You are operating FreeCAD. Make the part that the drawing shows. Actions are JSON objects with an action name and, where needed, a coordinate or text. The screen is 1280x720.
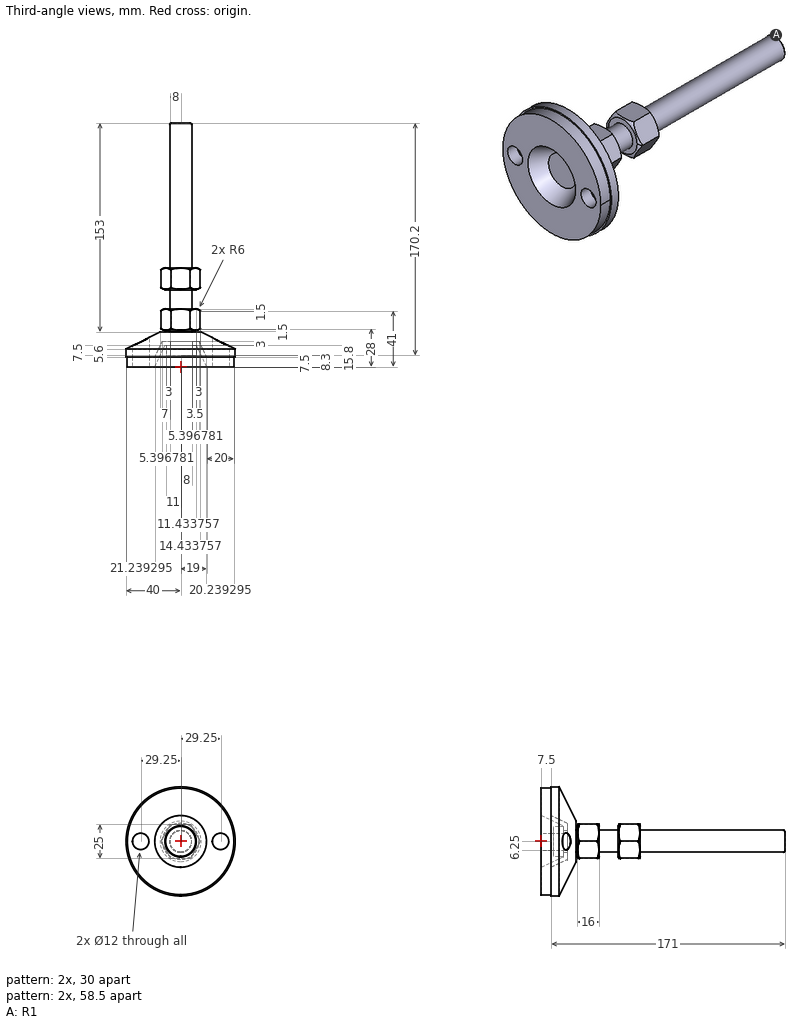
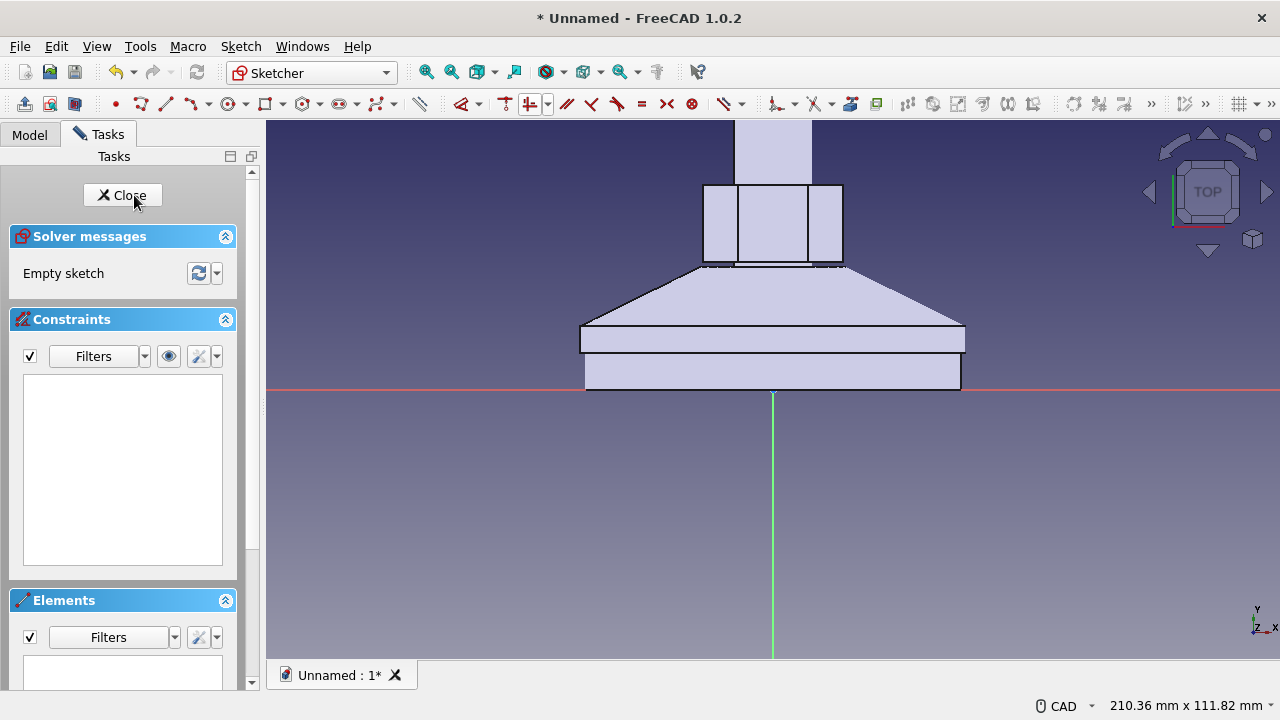
{"action": "left_click", "coordinate": [75, 104]}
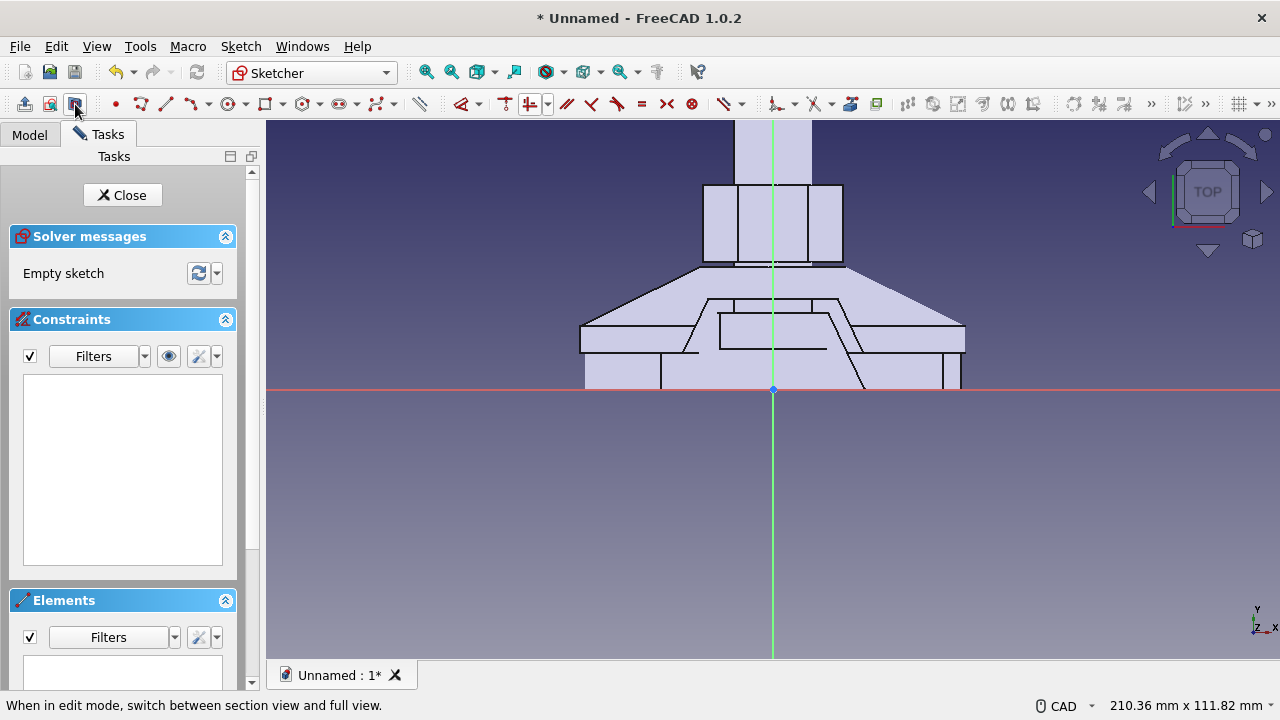
{"action": "scroll", "coordinate": [878, 169], "scroll_direction": "up", "scroll_amount": 7}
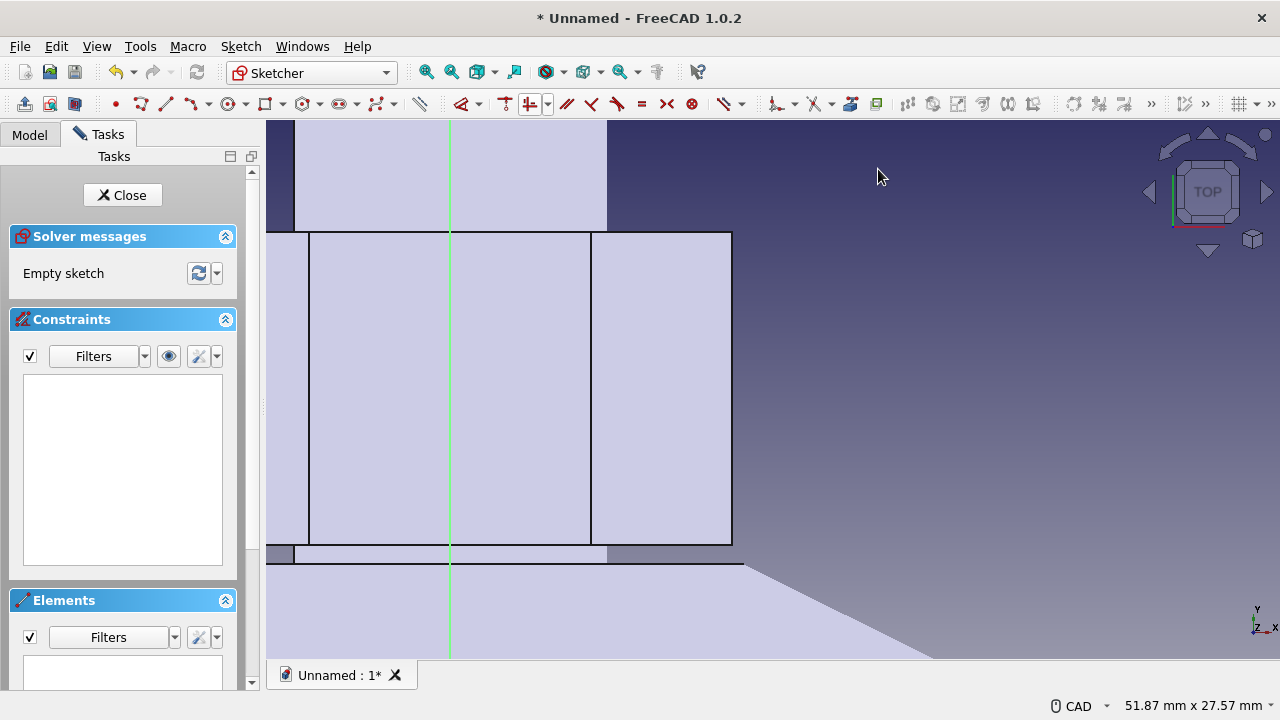
{"action": "left_click", "coordinate": [141, 104]}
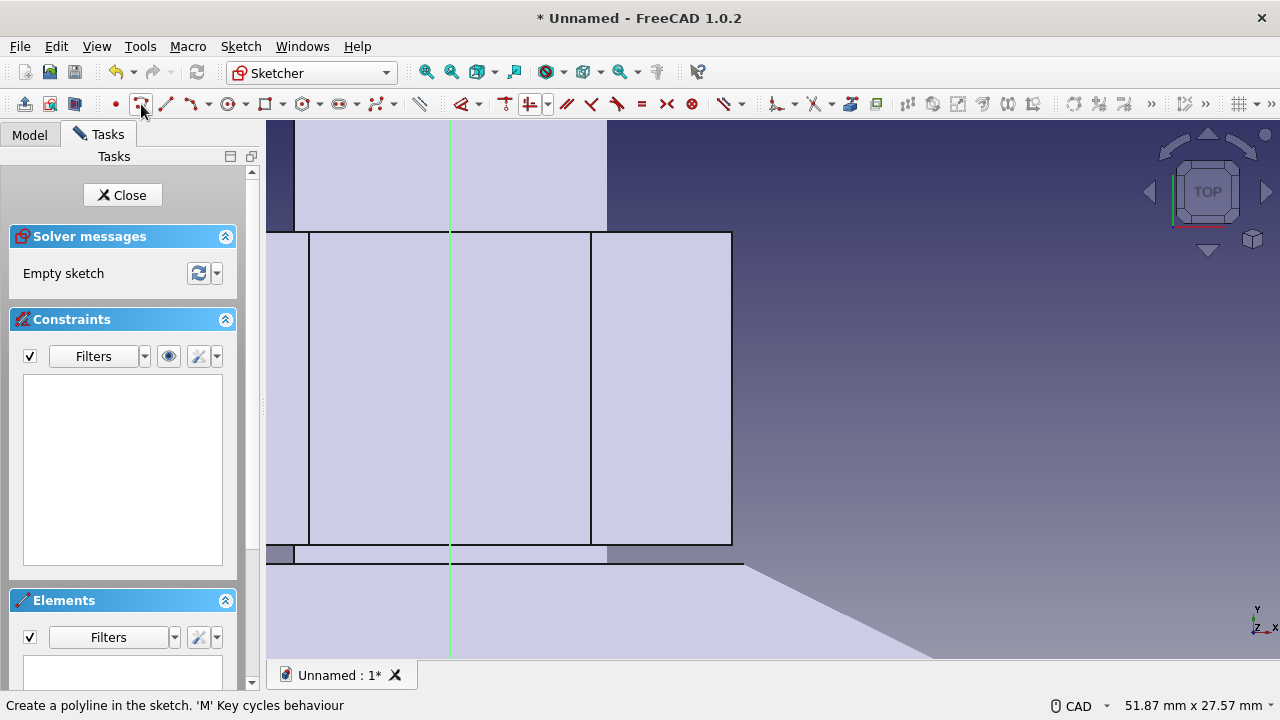
{"action": "left_click", "coordinate": [732, 261]}
{"action": "left_click", "coordinate": [732, 232]}
{"action": "left_click", "coordinate": [674, 232]}
{"action": "right_click", "coordinate": [674, 232]}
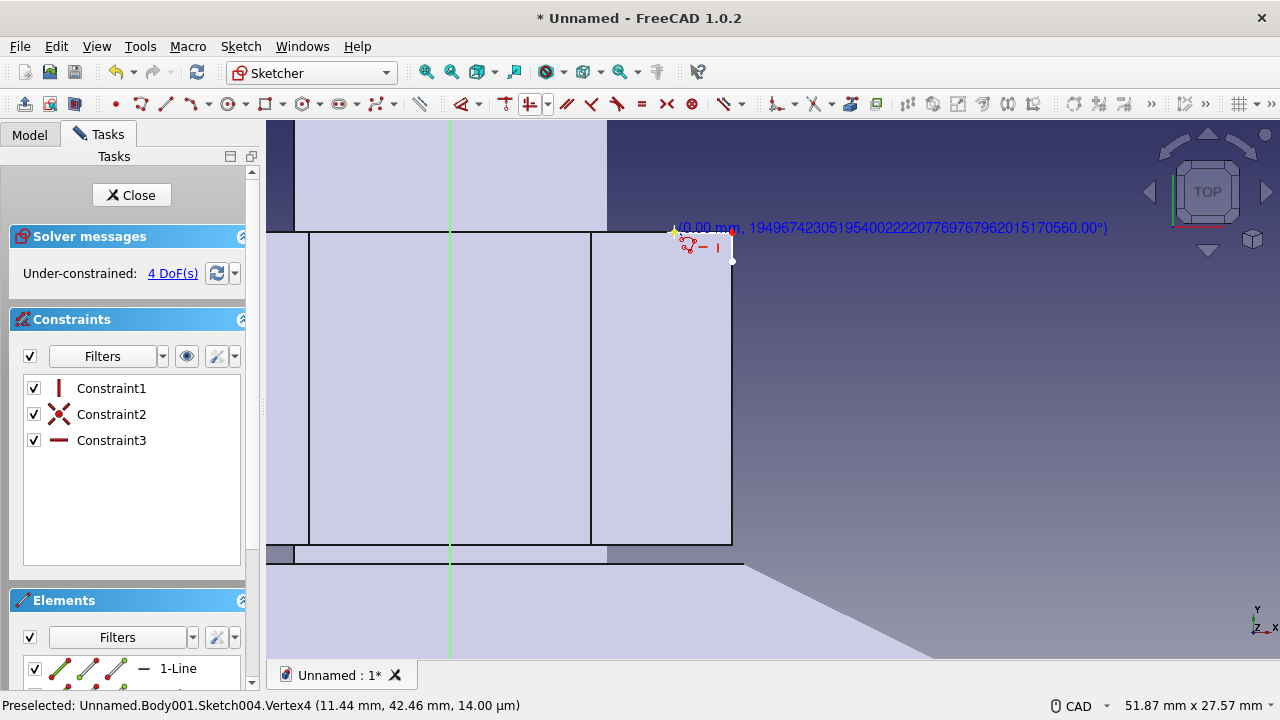
{"action": "left_click", "coordinate": [190, 104]}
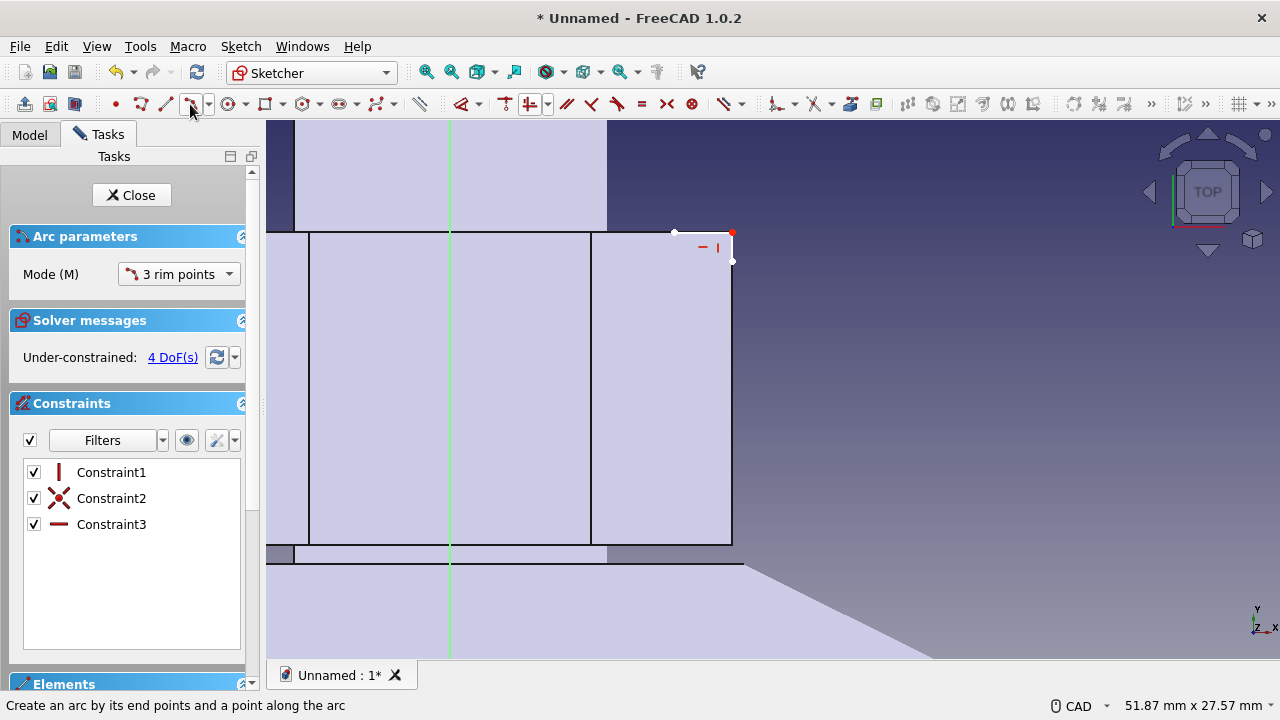
{"action": "left_click", "coordinate": [674, 233]}
{"action": "left_click", "coordinate": [732, 262]}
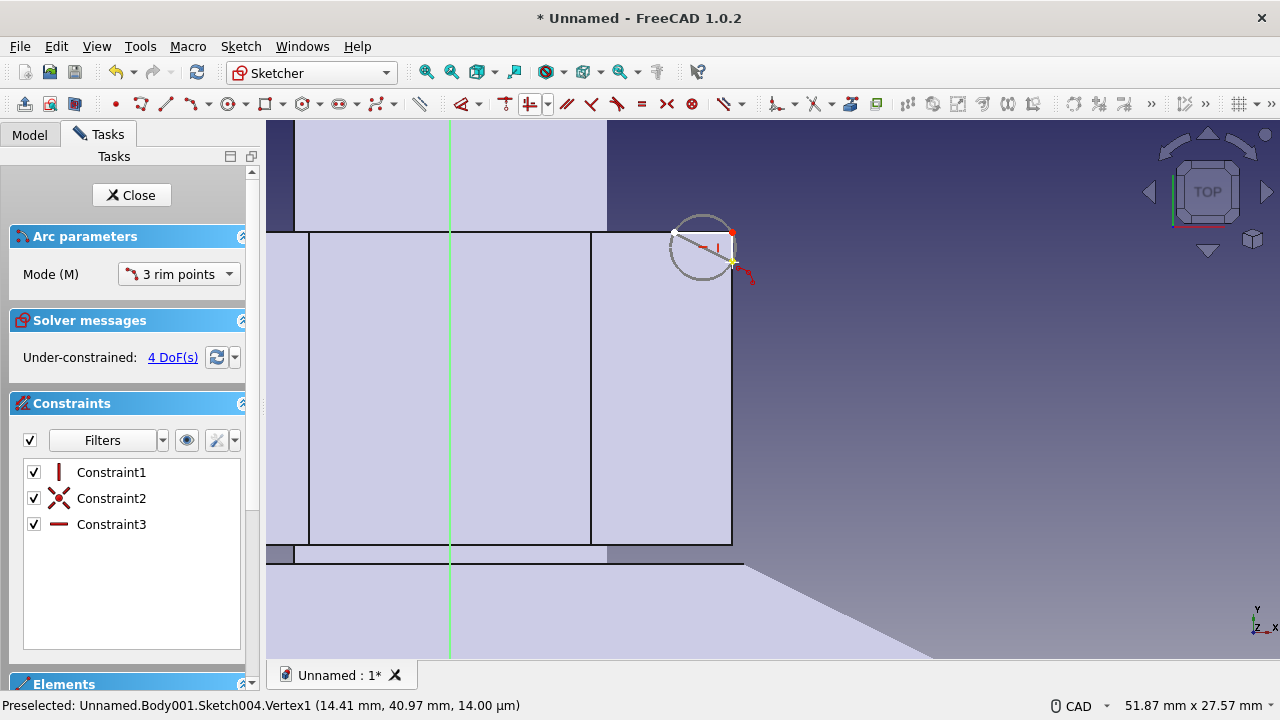
{"action": "scroll", "coordinate": [705, 243], "scroll_direction": "up", "scroll_amount": 7}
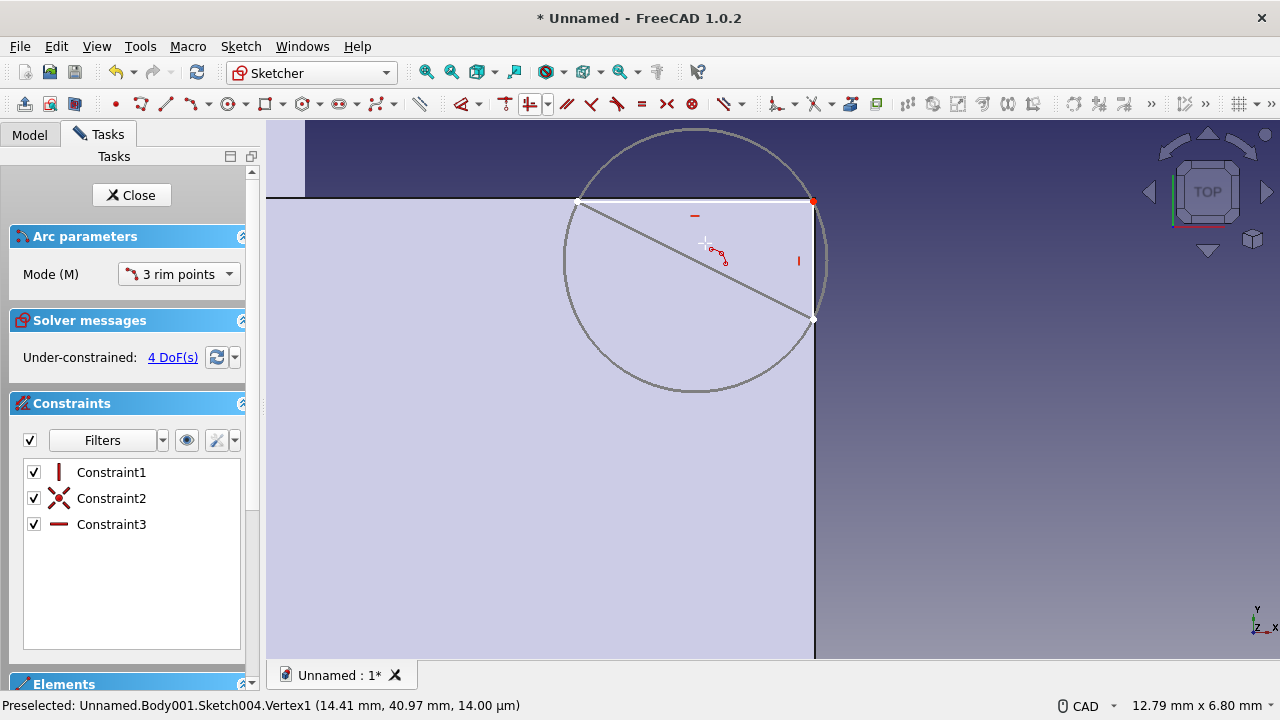
{"action": "left_click", "coordinate": [705, 241]}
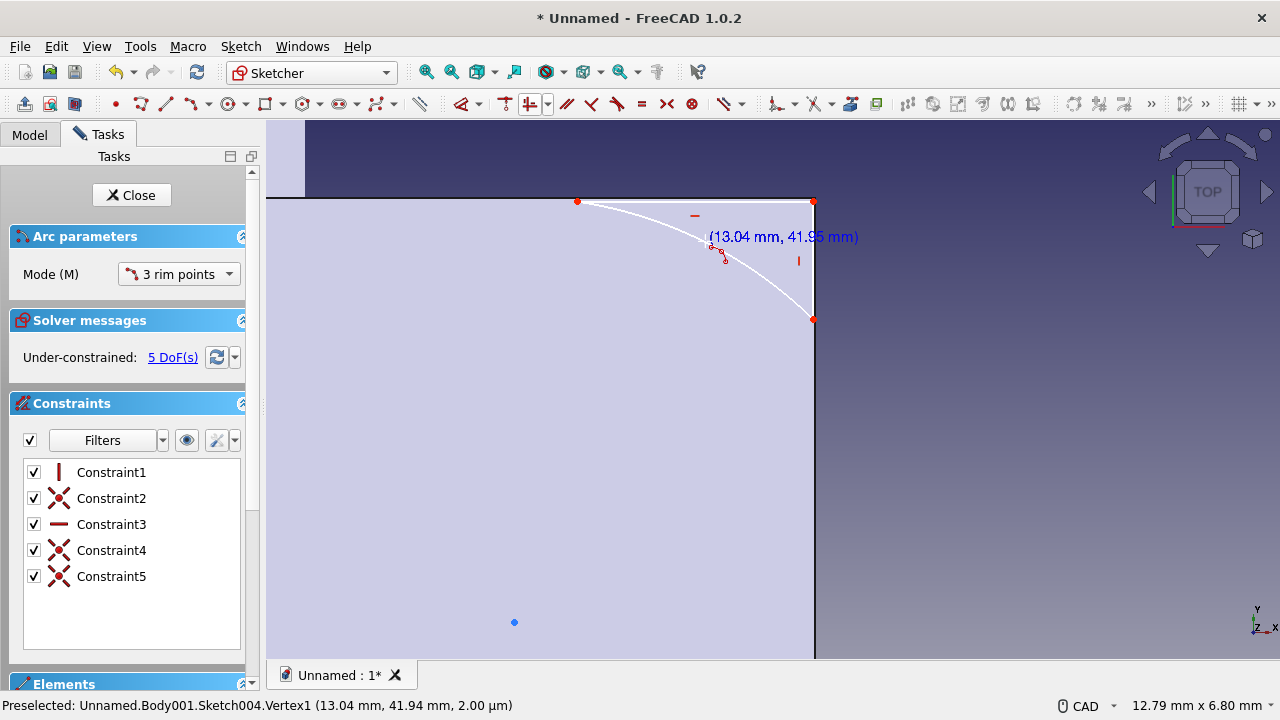
{"action": "left_click", "coordinate": [141, 104]}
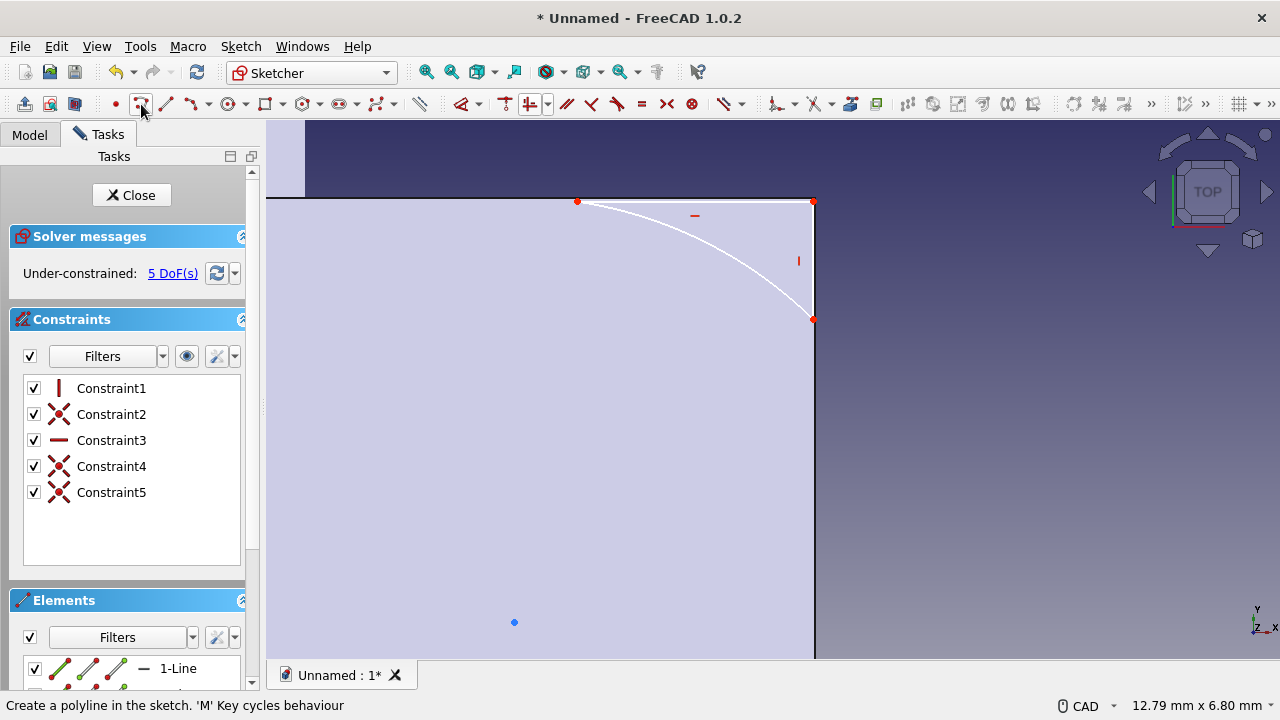
{"action": "scroll", "coordinate": [707, 245], "scroll_direction": "down", "scroll_amount": 7}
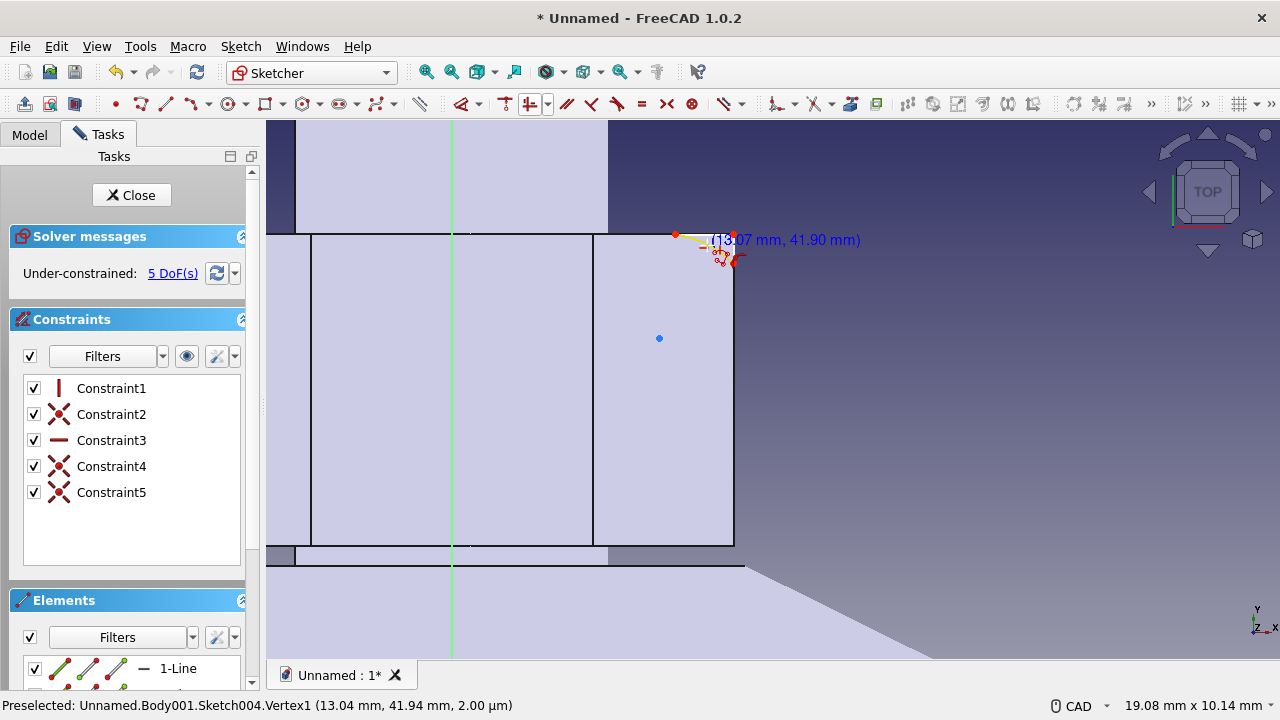
{"action": "left_click", "coordinate": [675, 546]}
{"action": "left_click", "coordinate": [734, 546]}
{"action": "left_click", "coordinate": [734, 517]}
{"action": "right_click", "coordinate": [734, 517]}